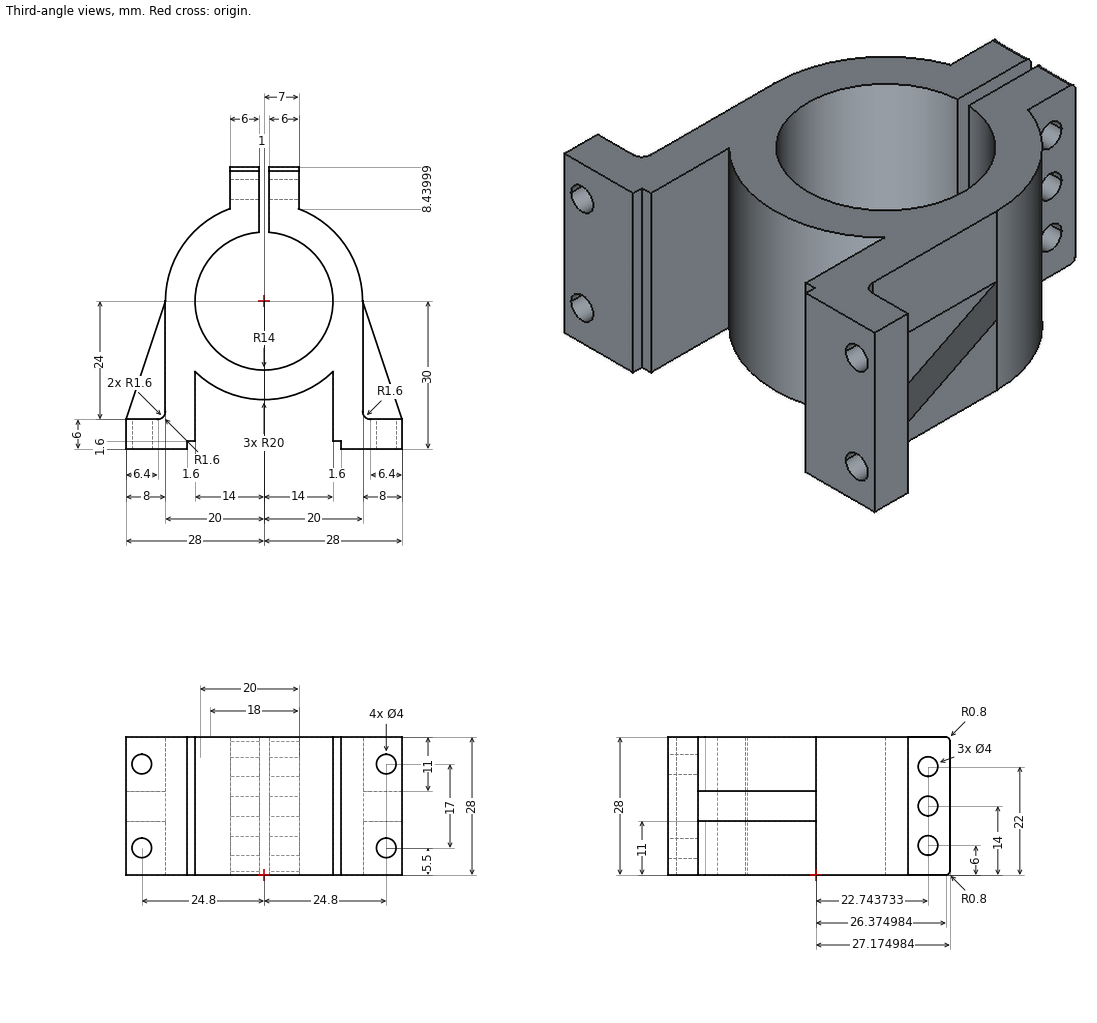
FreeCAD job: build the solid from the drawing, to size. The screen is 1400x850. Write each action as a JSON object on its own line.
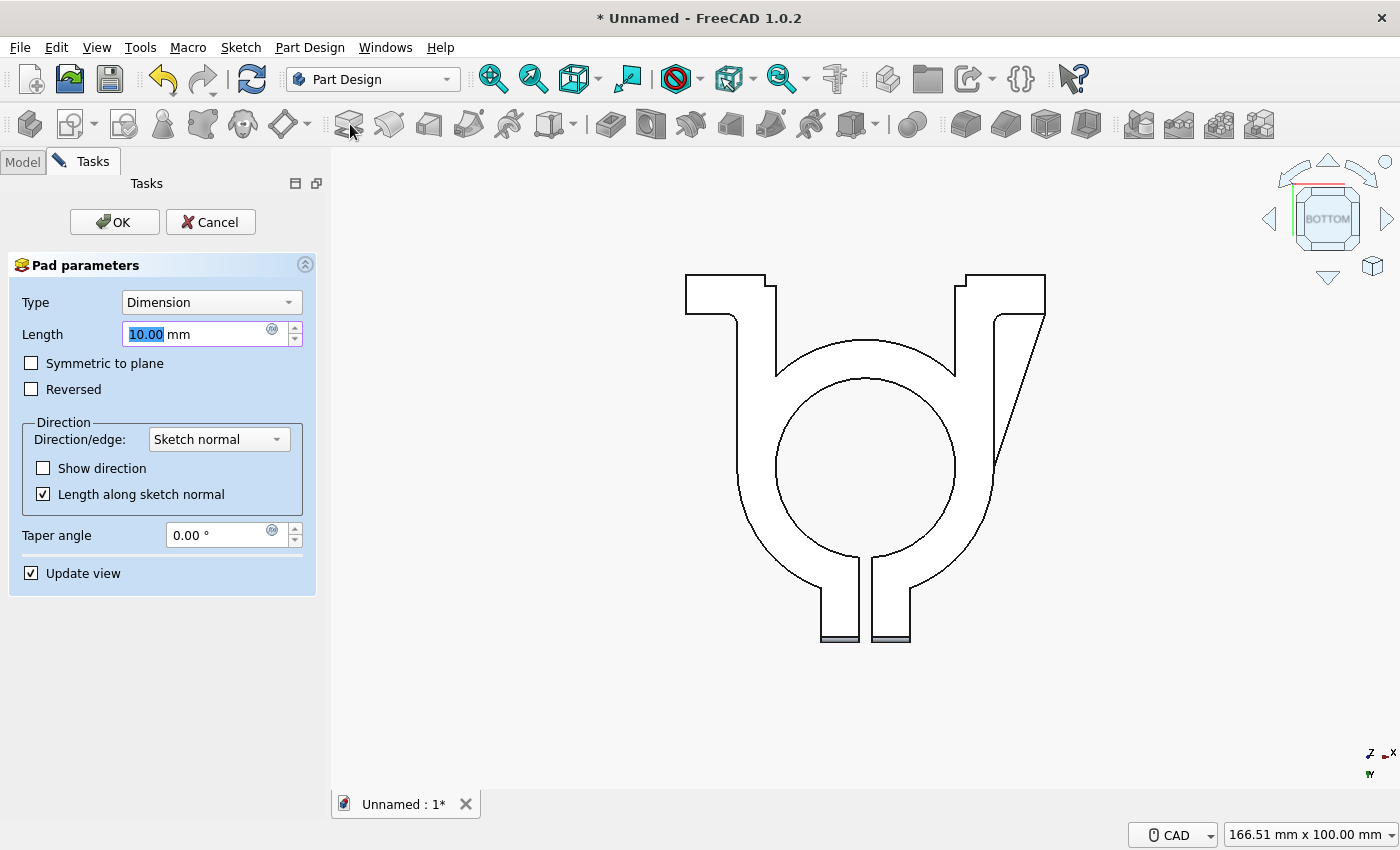
{"action": "type", "text": "28"}
{"action": "key", "text": "Tab"}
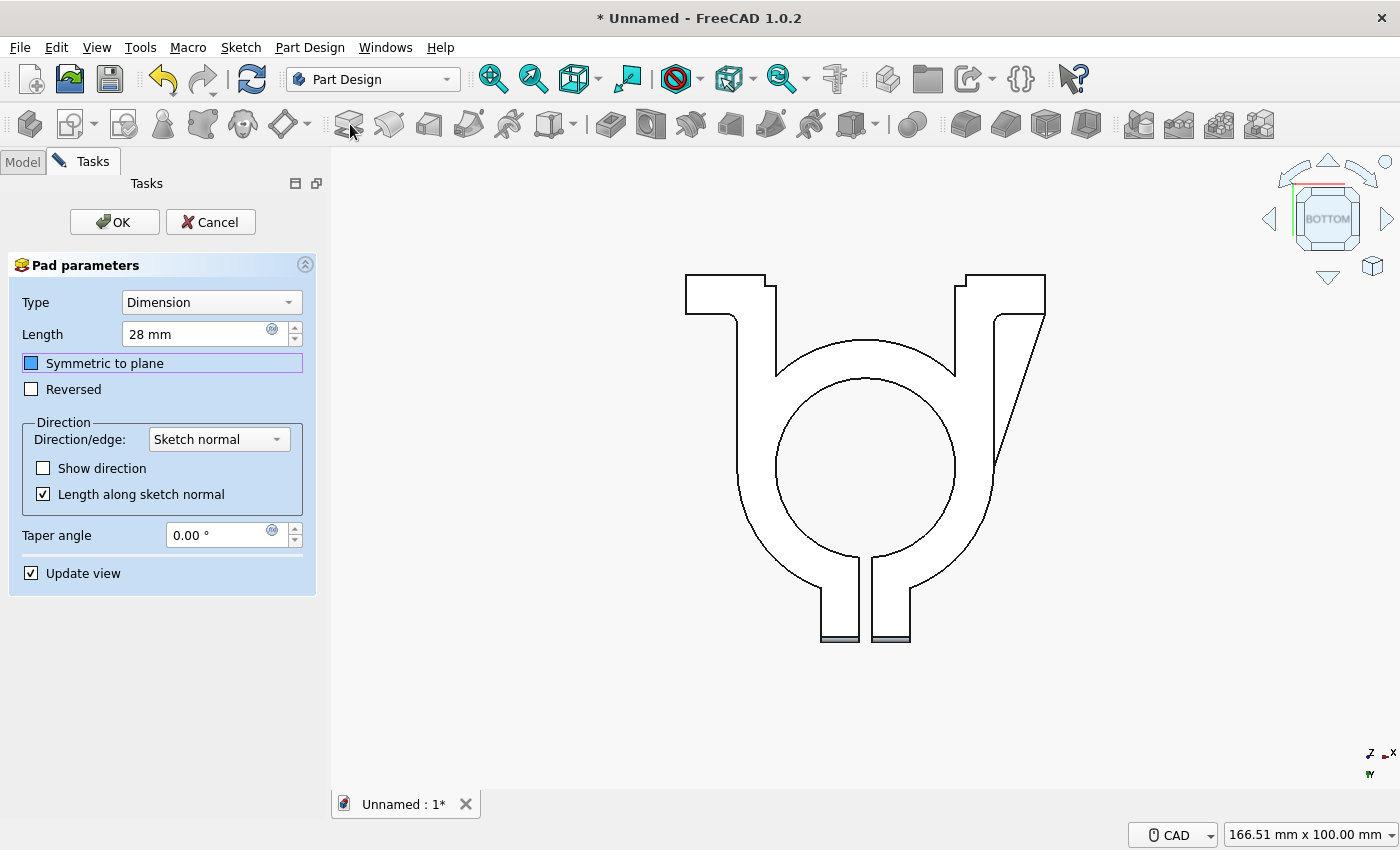
{"action": "left_click", "coordinate": [30, 389]}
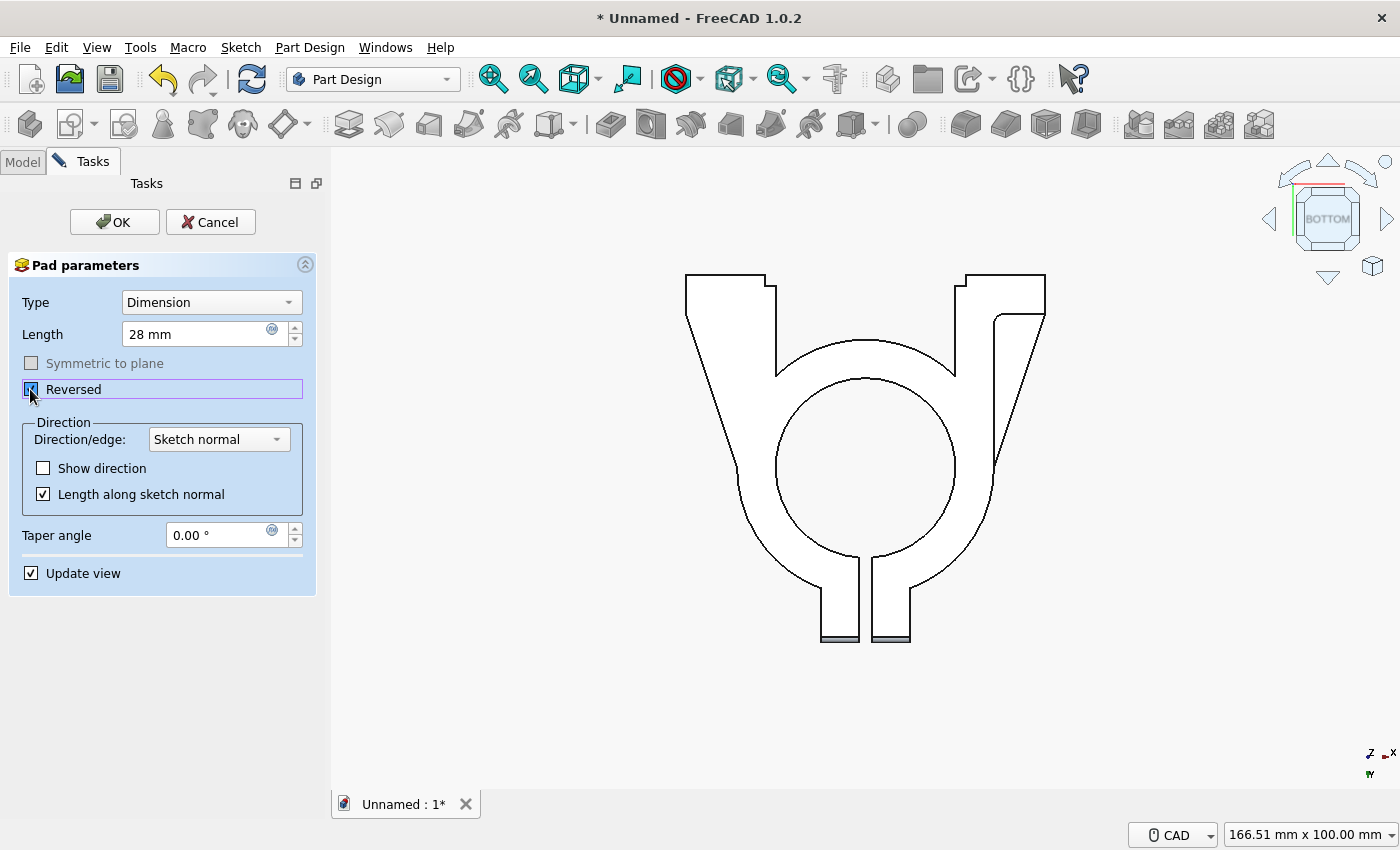
{"action": "left_click", "coordinate": [115, 222]}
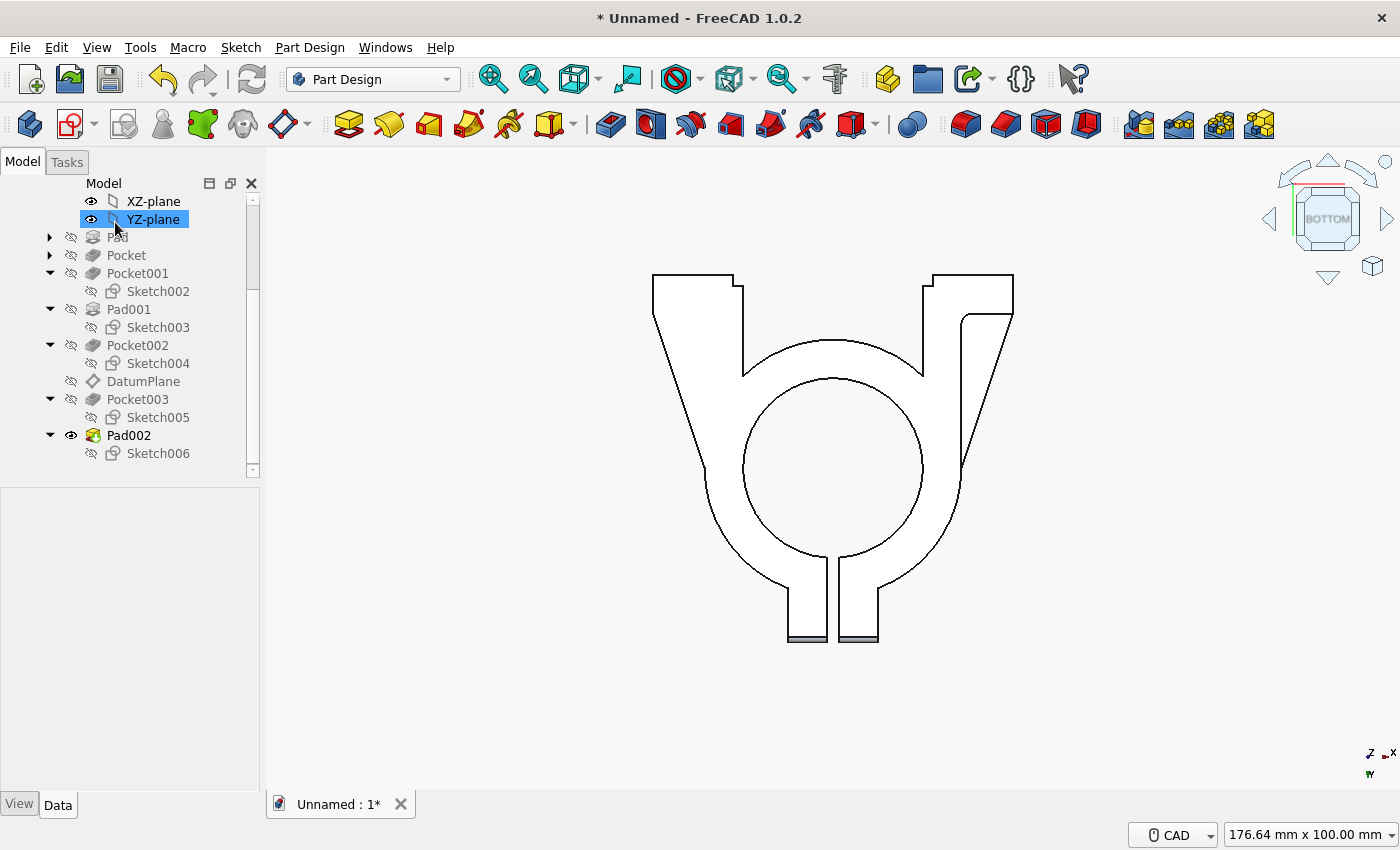
{"action": "left_click", "coordinate": [70, 124]}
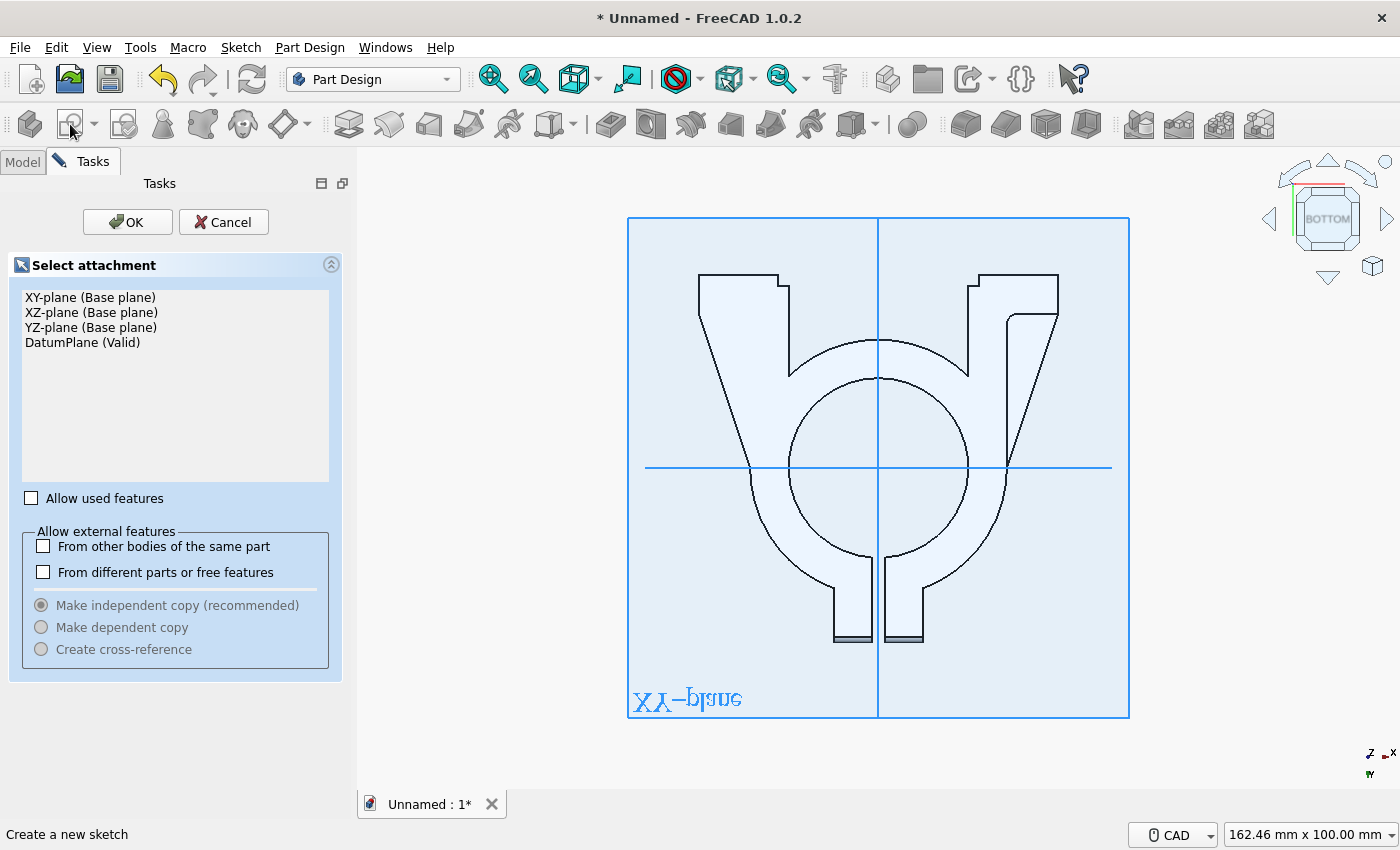
{"action": "left_click", "coordinate": [82, 298]}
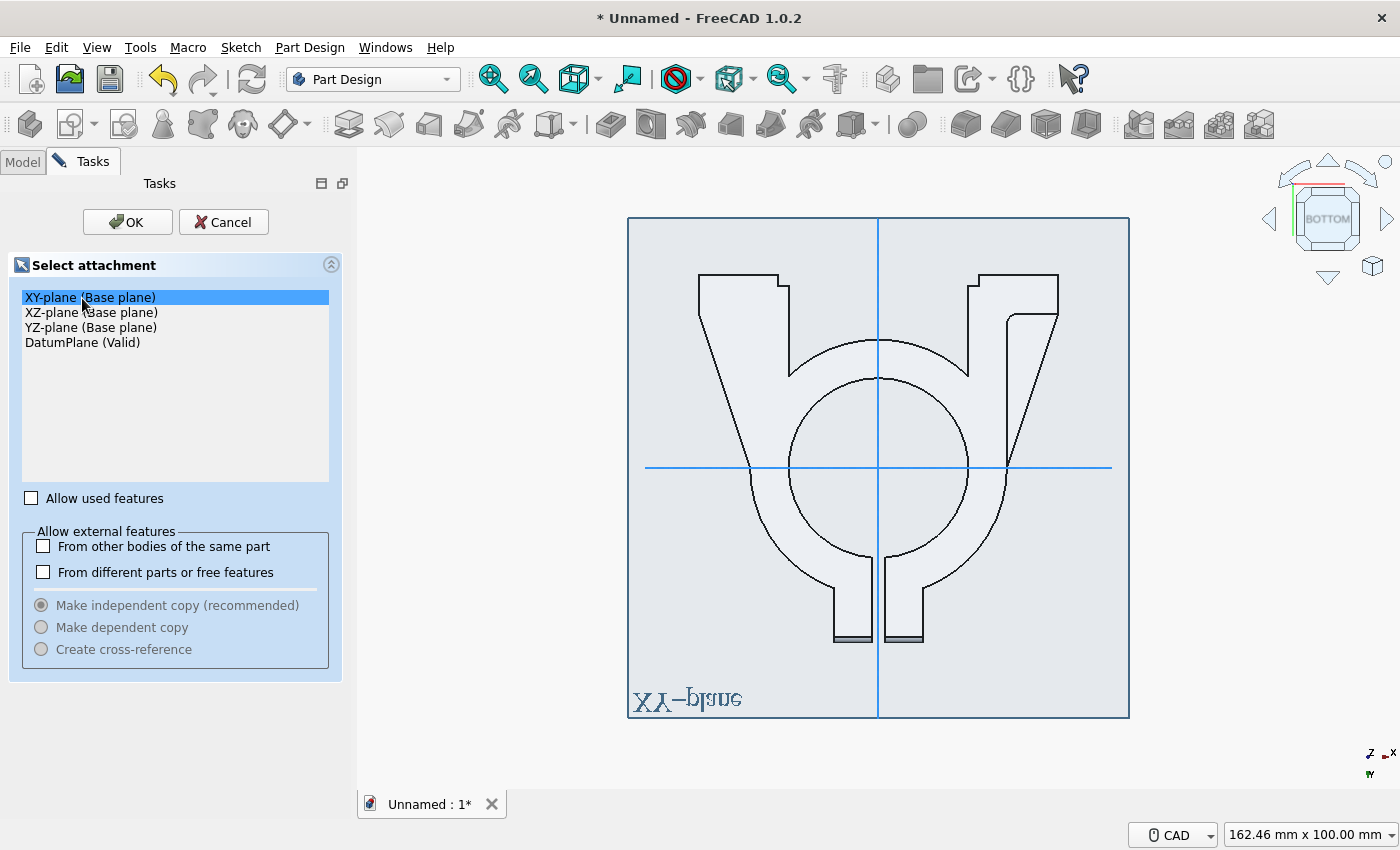
{"action": "left_click", "coordinate": [128, 222]}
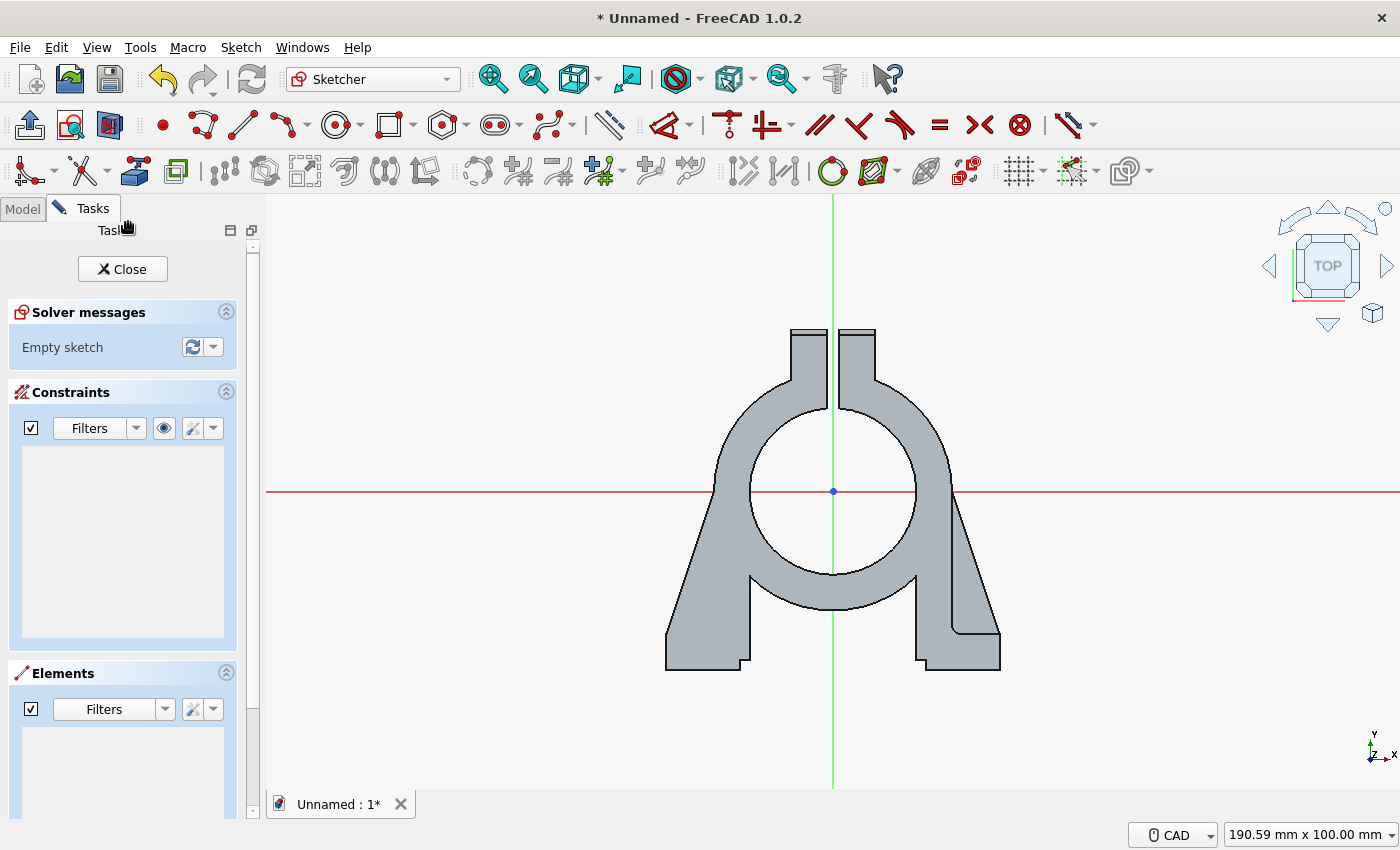
{"action": "left_click", "coordinate": [110, 126]}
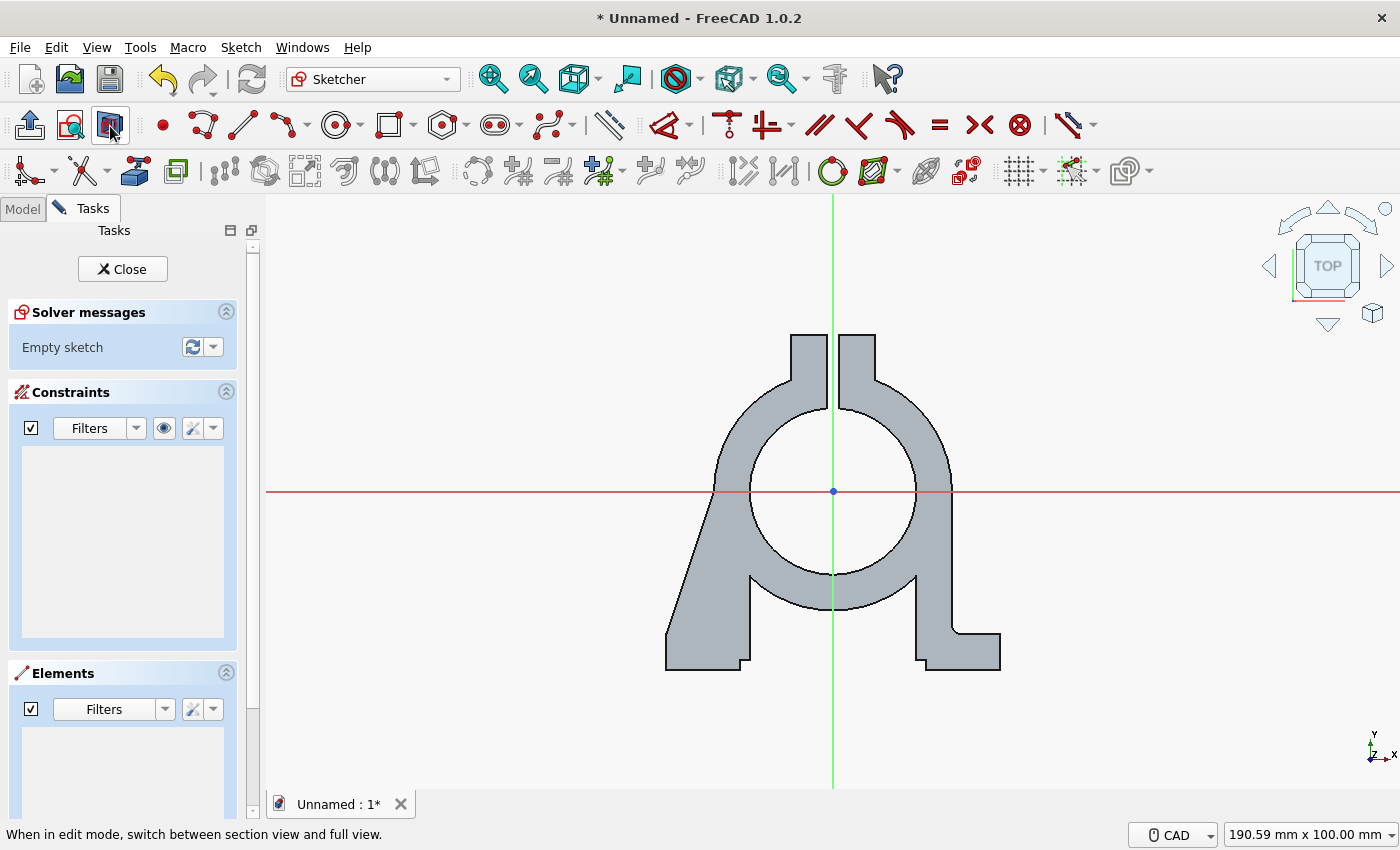
{"action": "scroll", "coordinate": [741, 604], "scroll_direction": "up", "scroll_amount": 5}